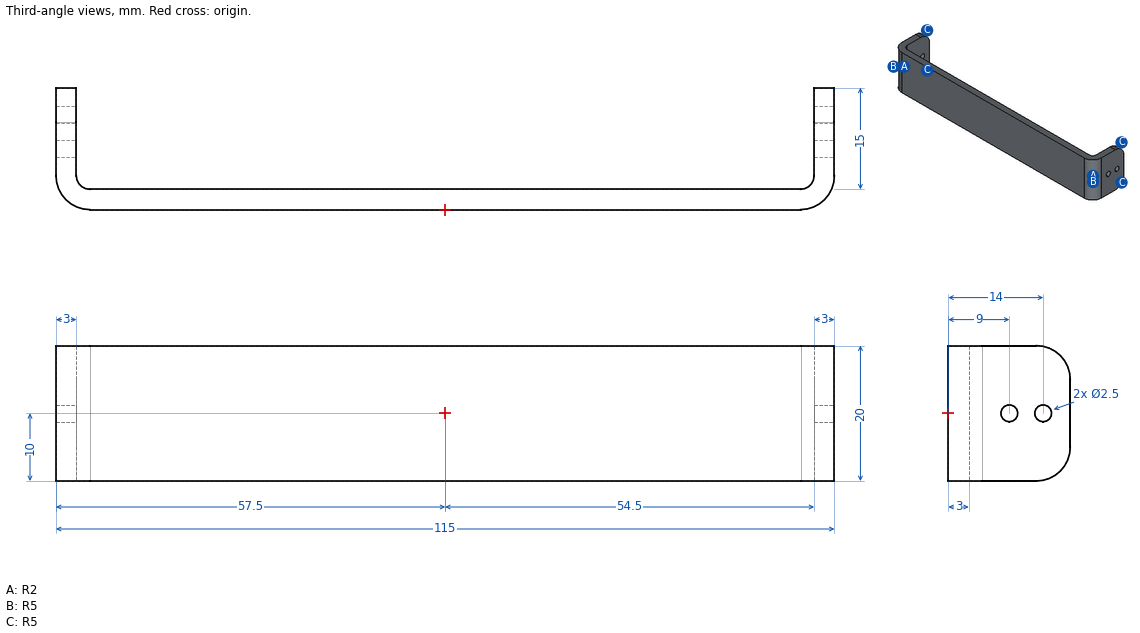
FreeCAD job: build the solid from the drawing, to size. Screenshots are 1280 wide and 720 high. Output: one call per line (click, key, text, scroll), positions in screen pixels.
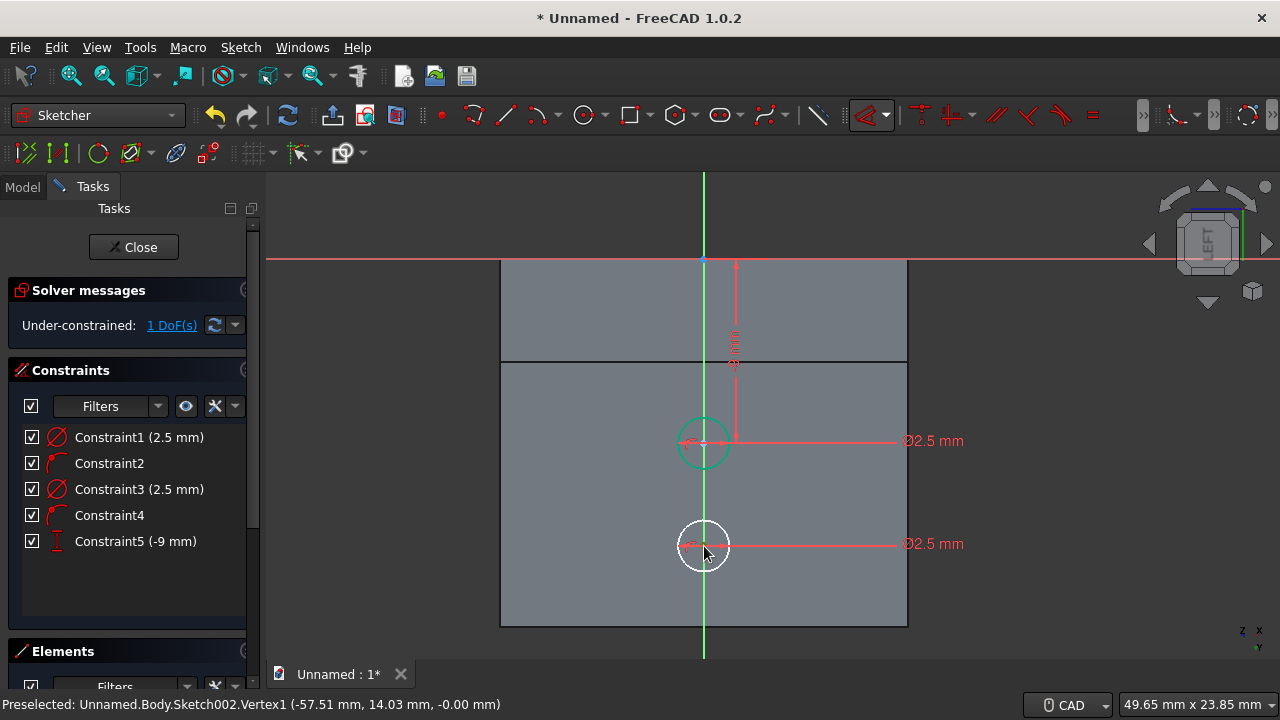
key(i)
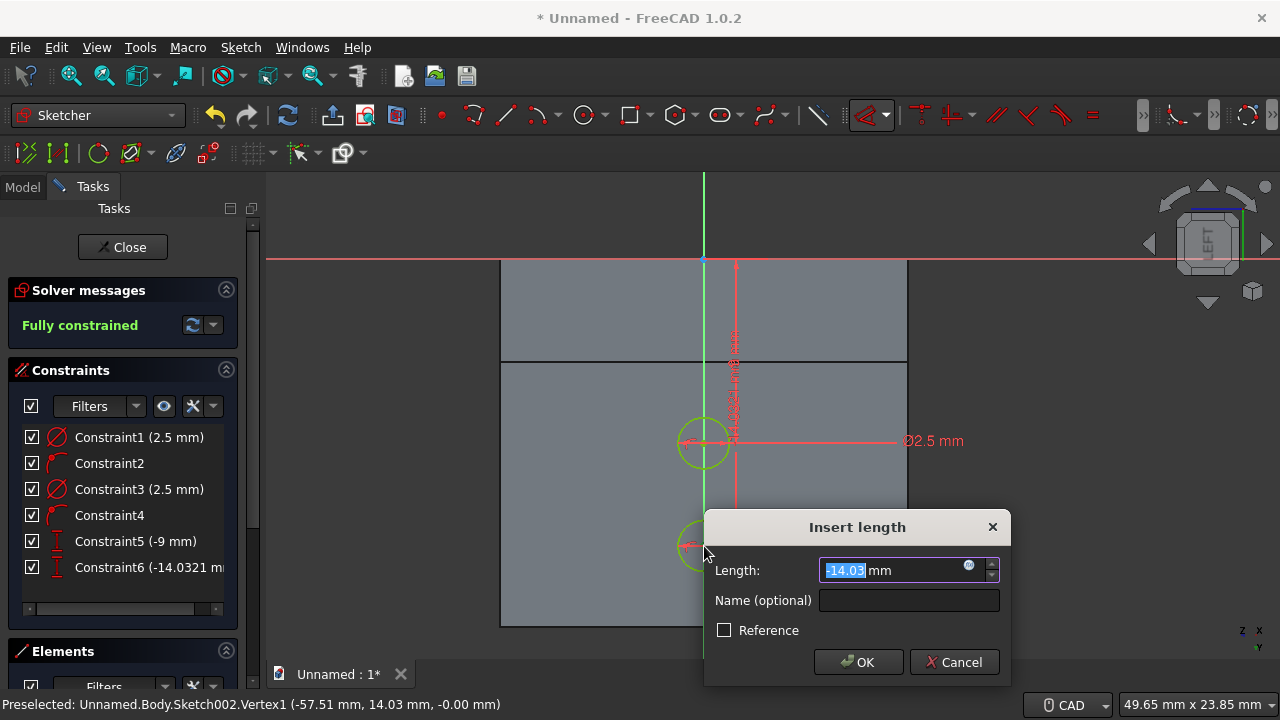
text(-14)
key(Return)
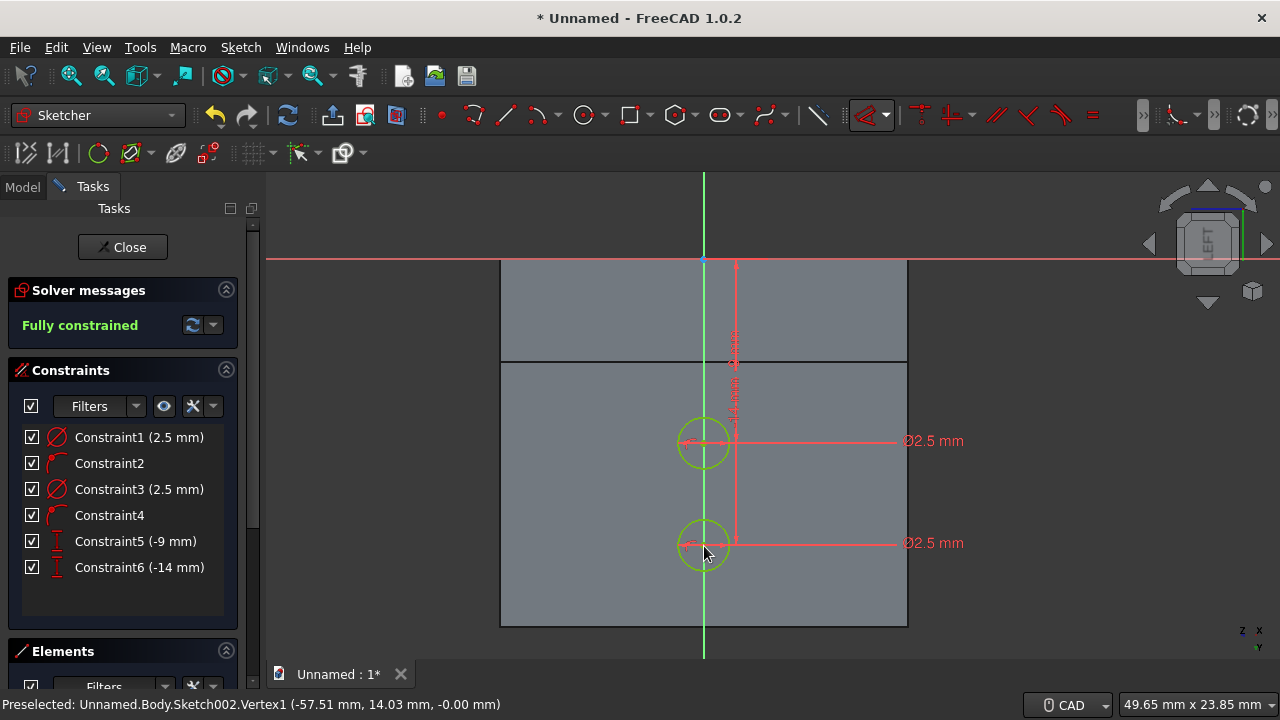
click(123, 247)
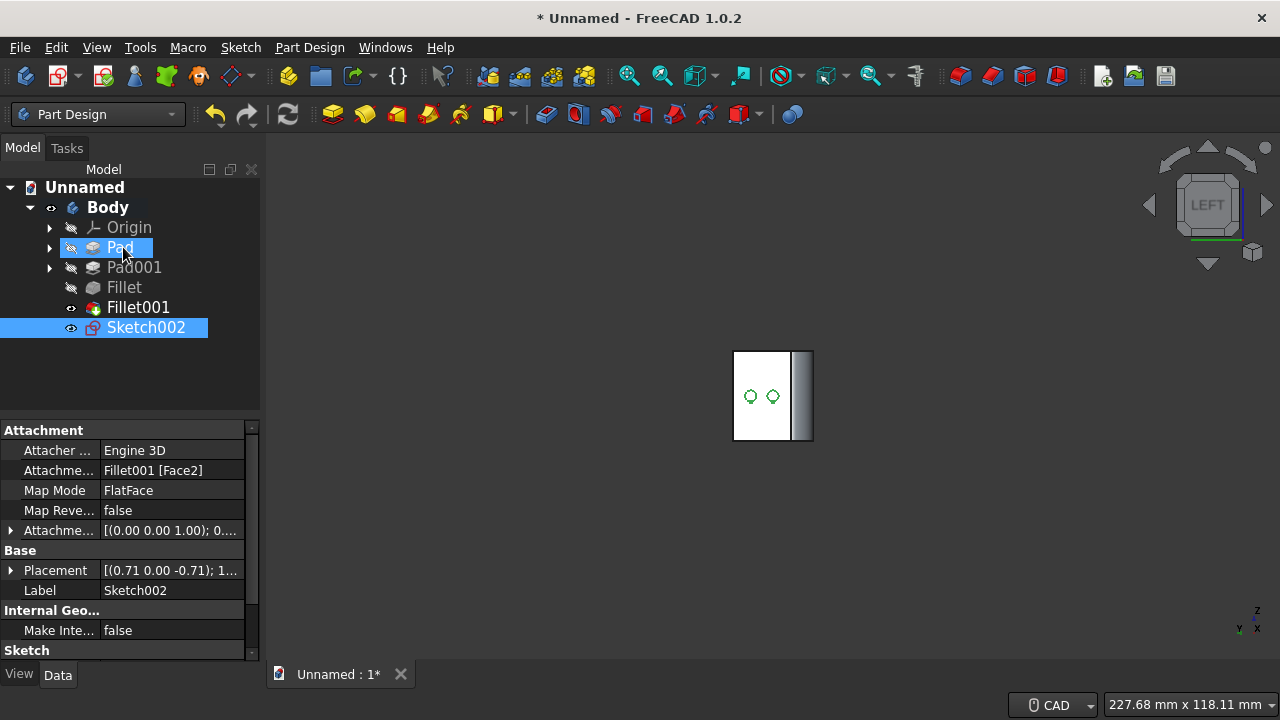
click(548, 114)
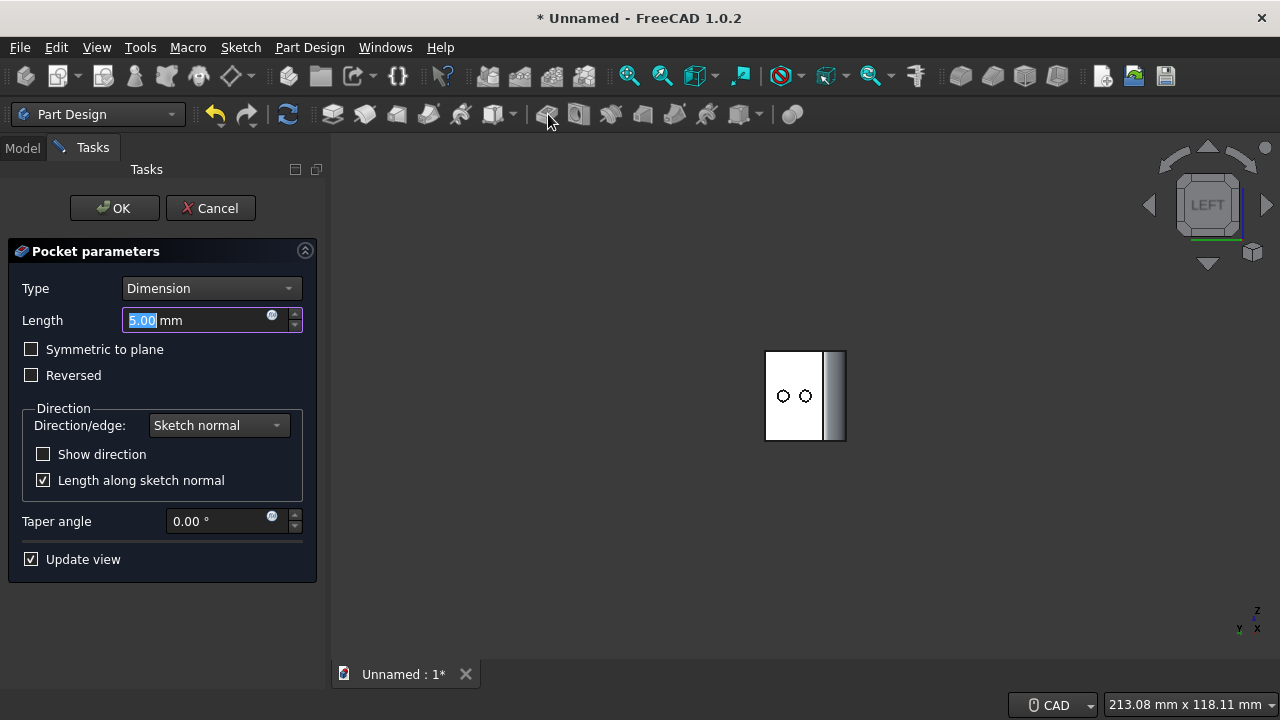
click(212, 288)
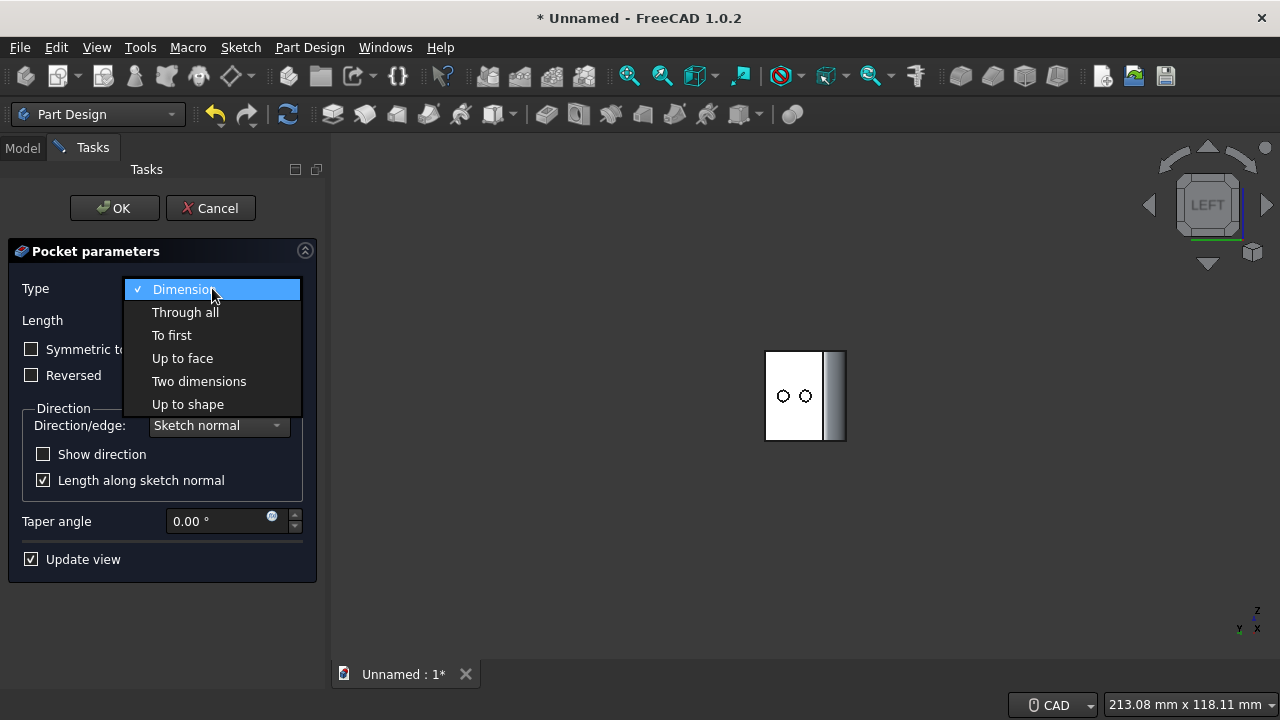
click(212, 312)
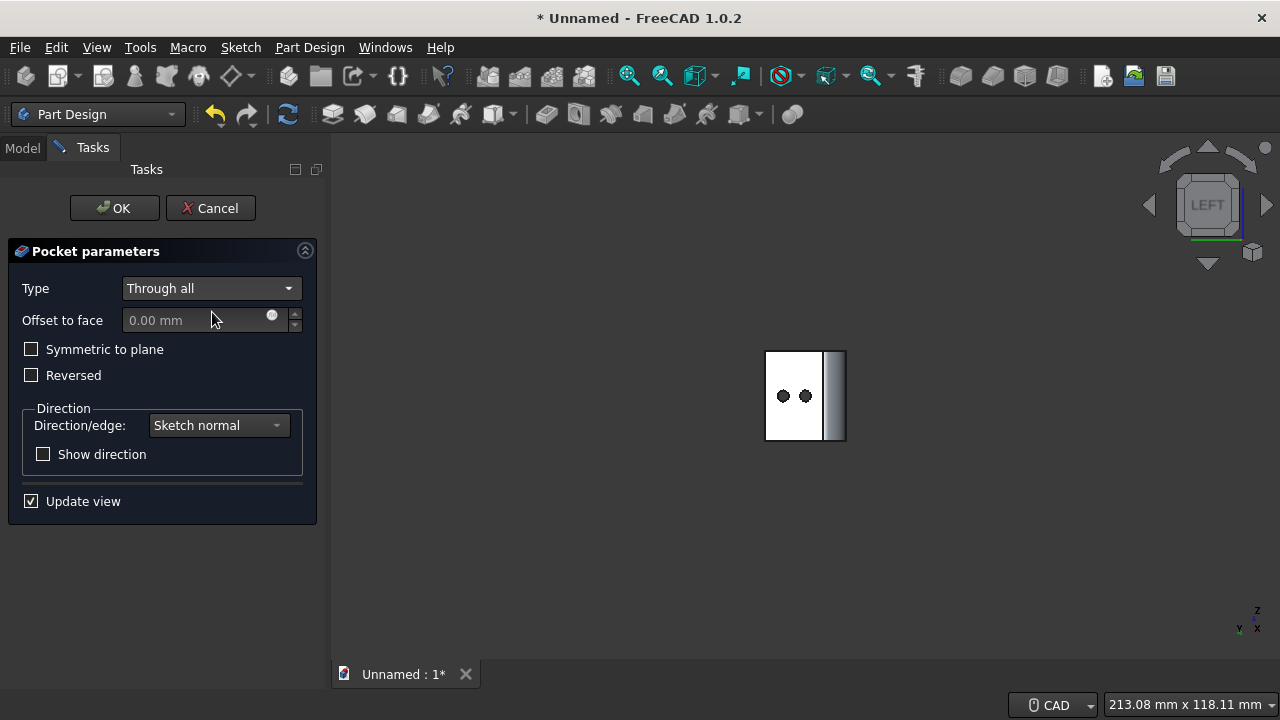
click(115, 208)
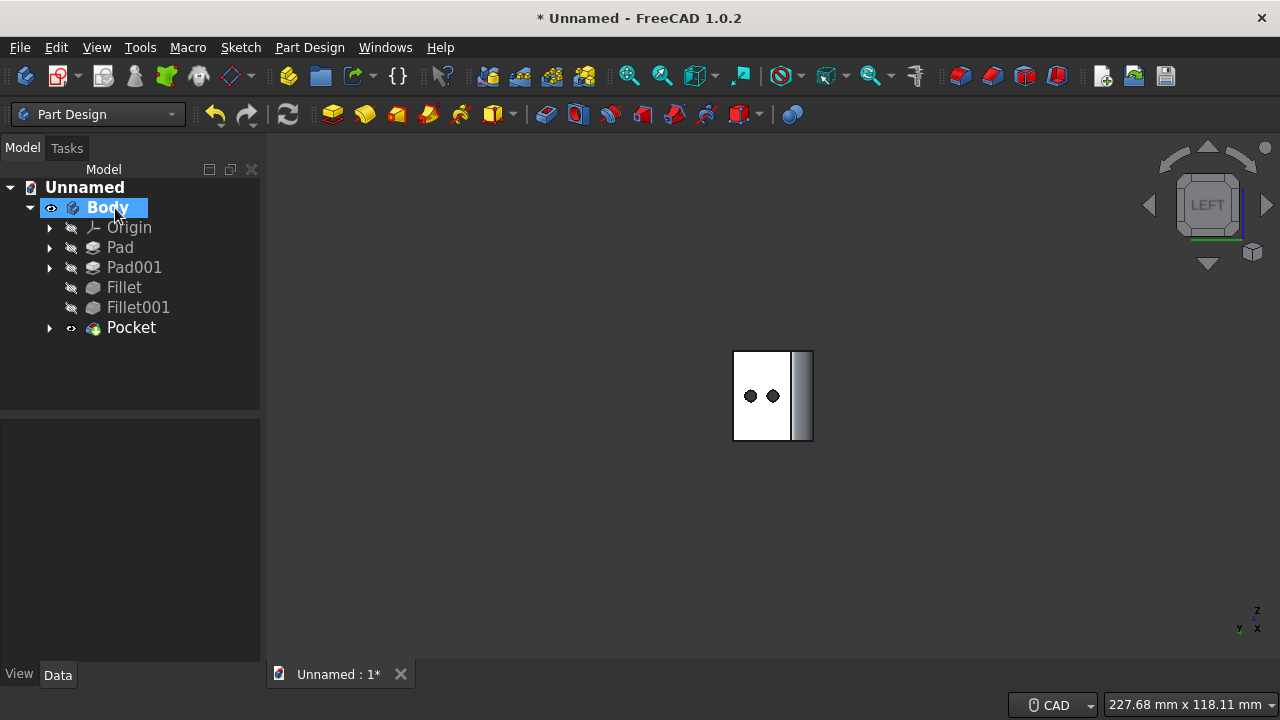
click(630, 76)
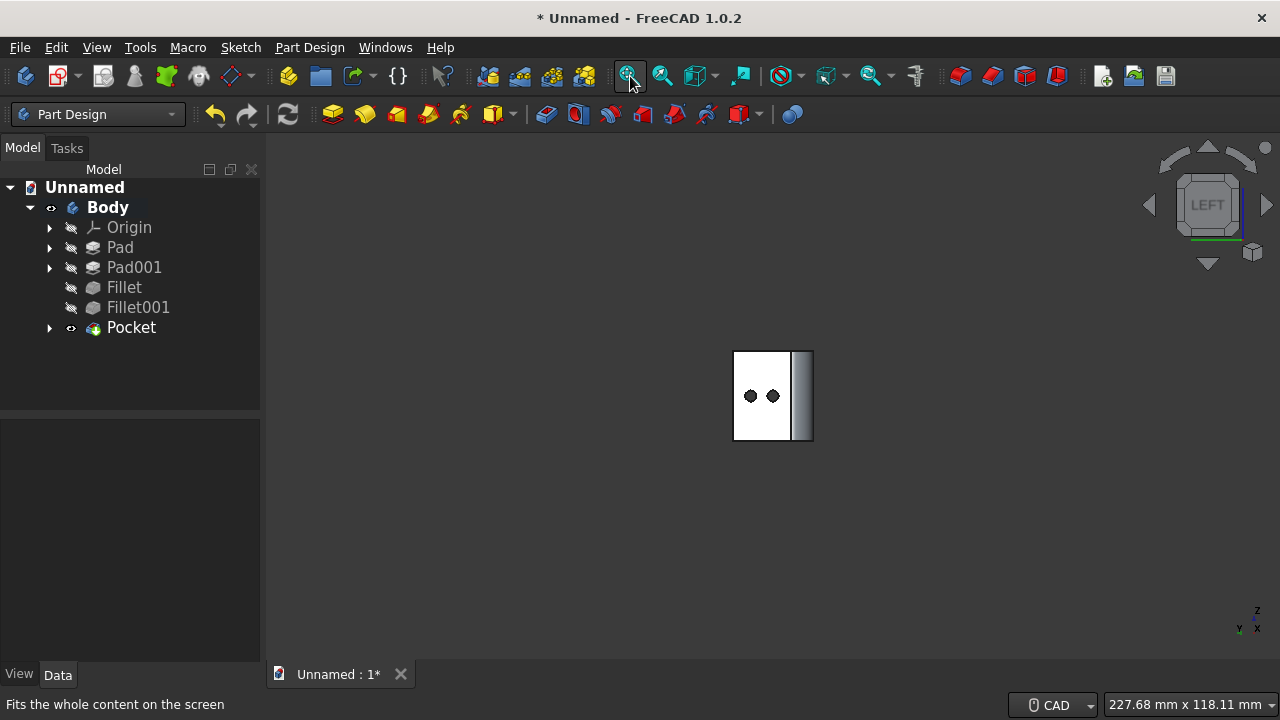
scroll(733, 350, up, 6)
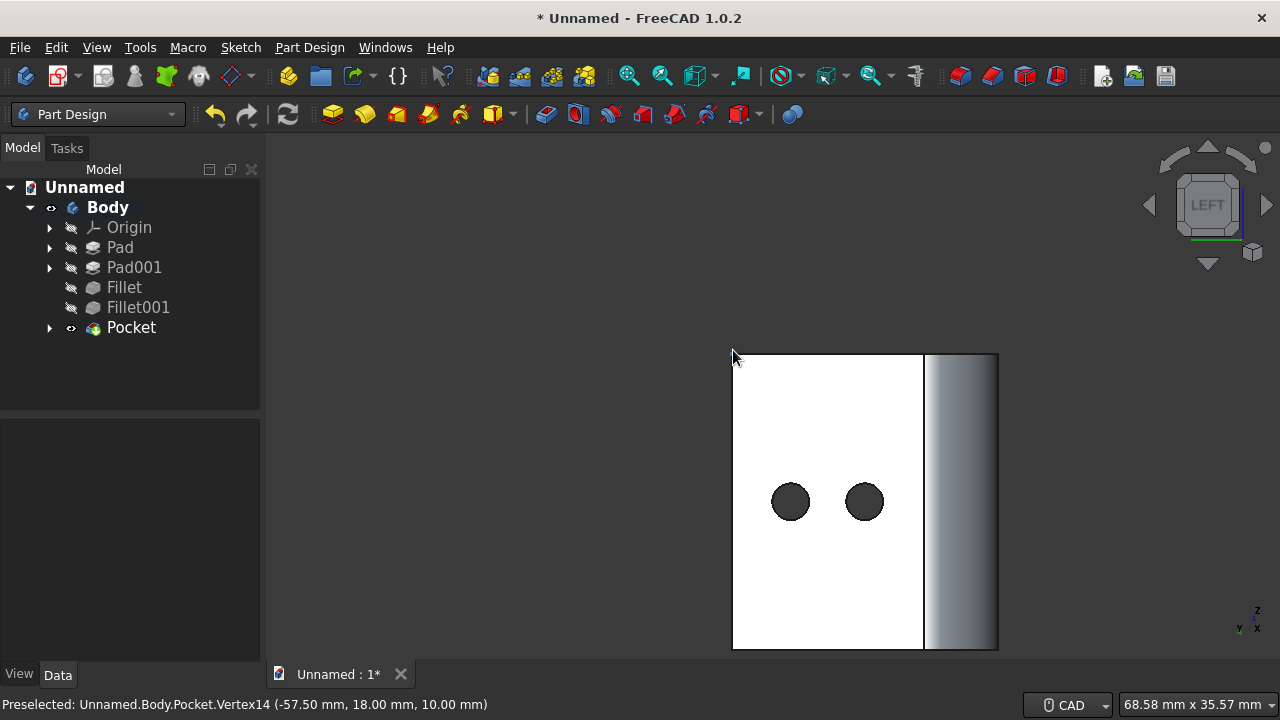
click(630, 76)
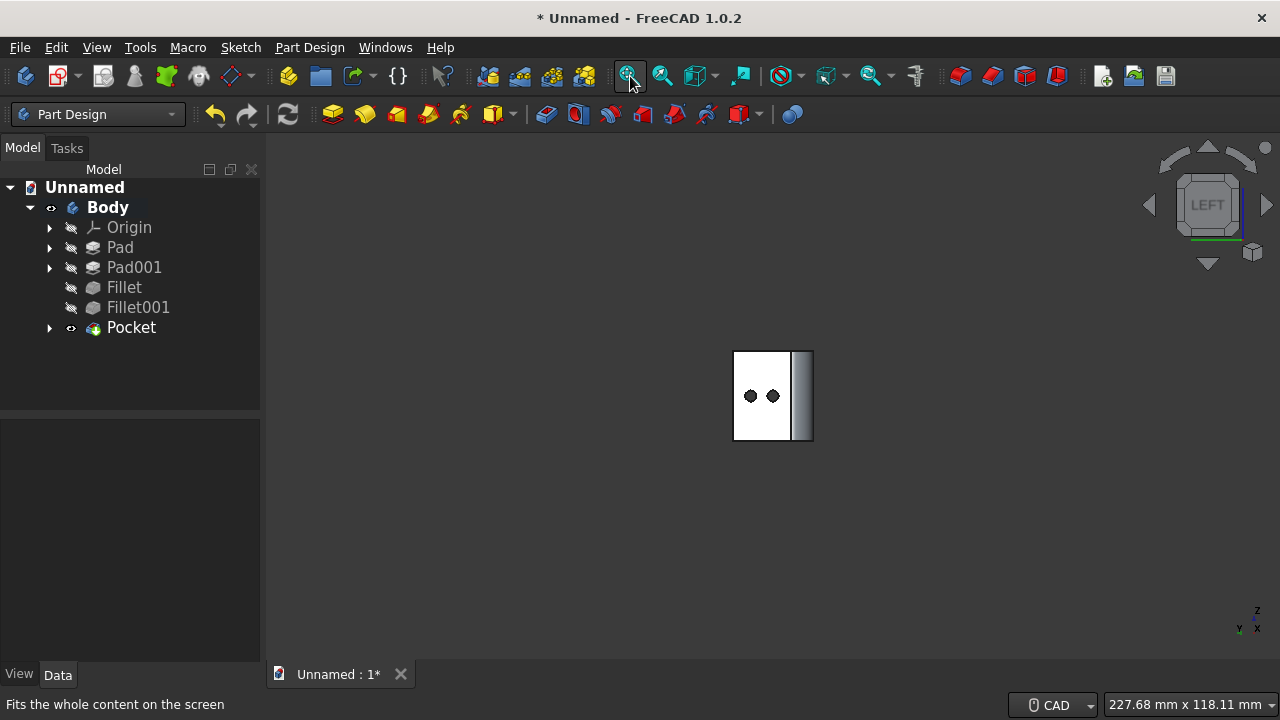
key(0)